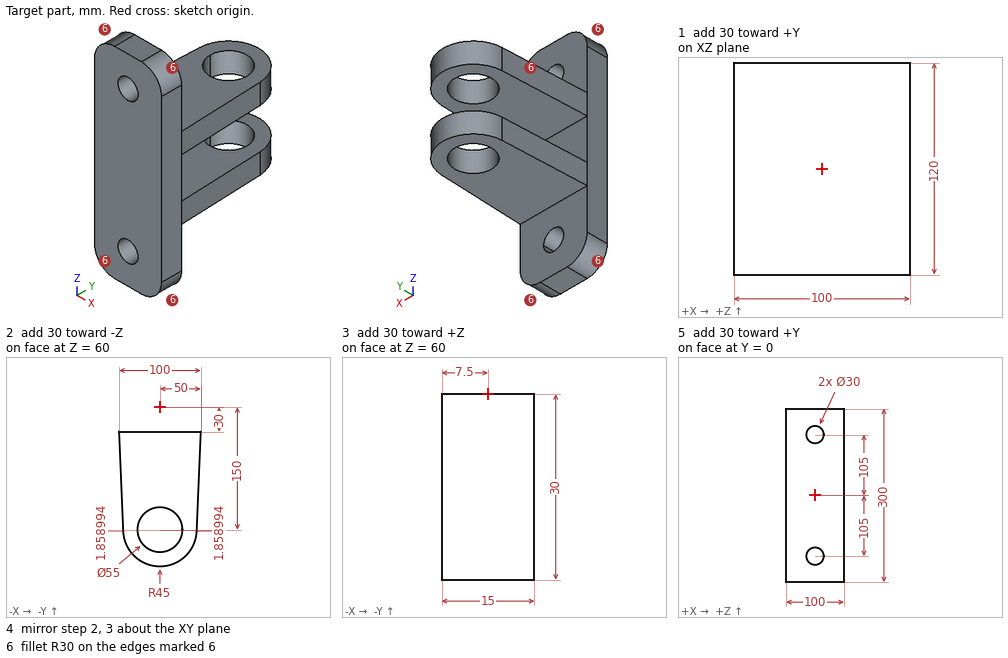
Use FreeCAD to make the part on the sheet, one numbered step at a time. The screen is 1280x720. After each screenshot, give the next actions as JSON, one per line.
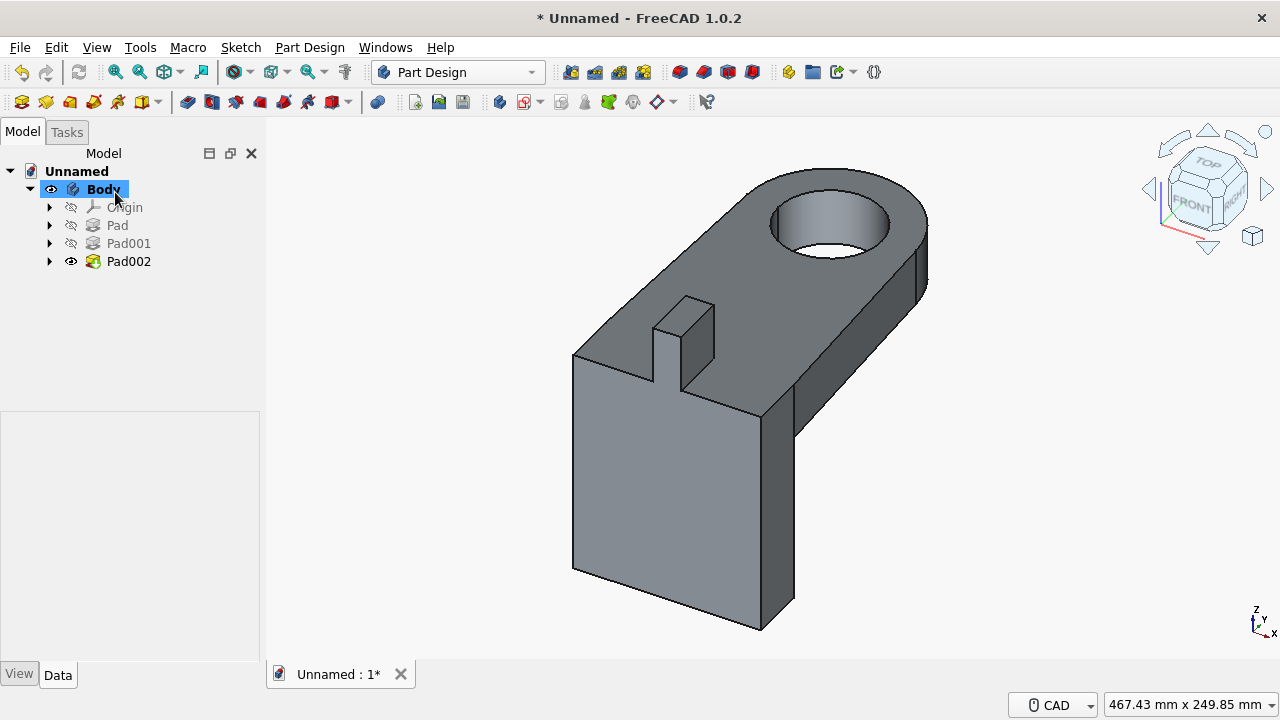
{"action": "key", "text": "v f"}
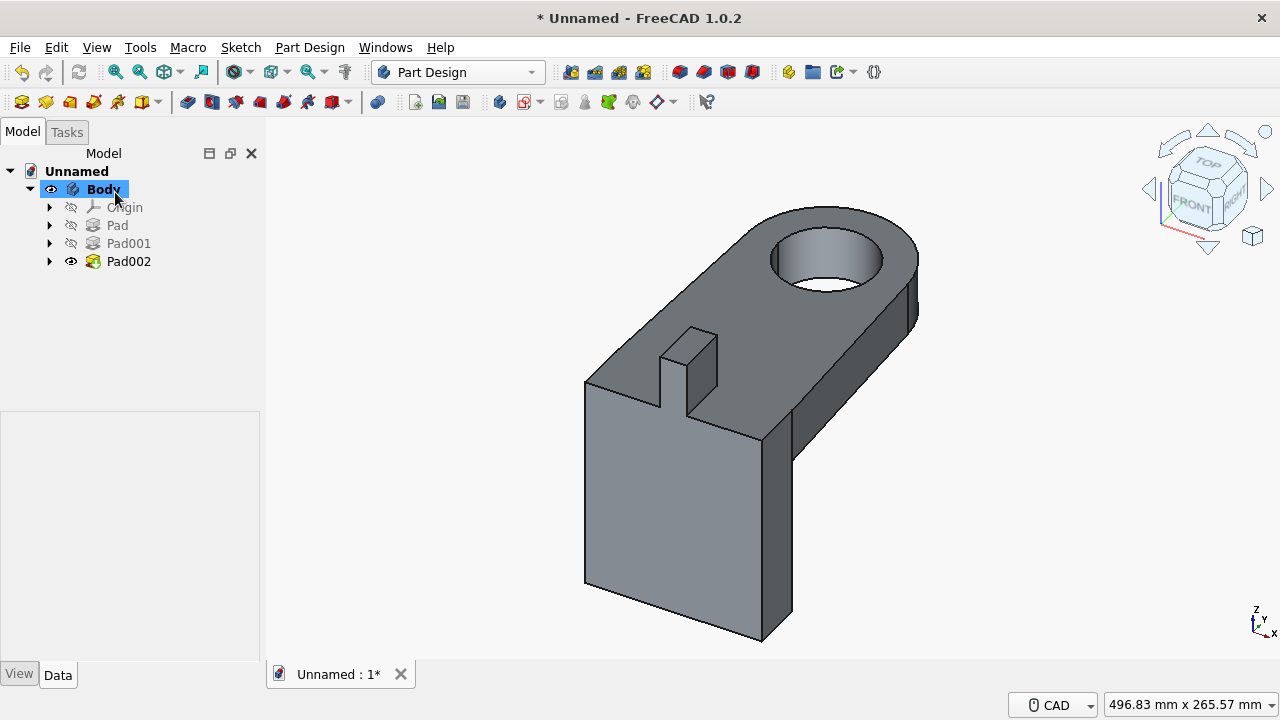
{"action": "left_click", "coordinate": [116, 243]}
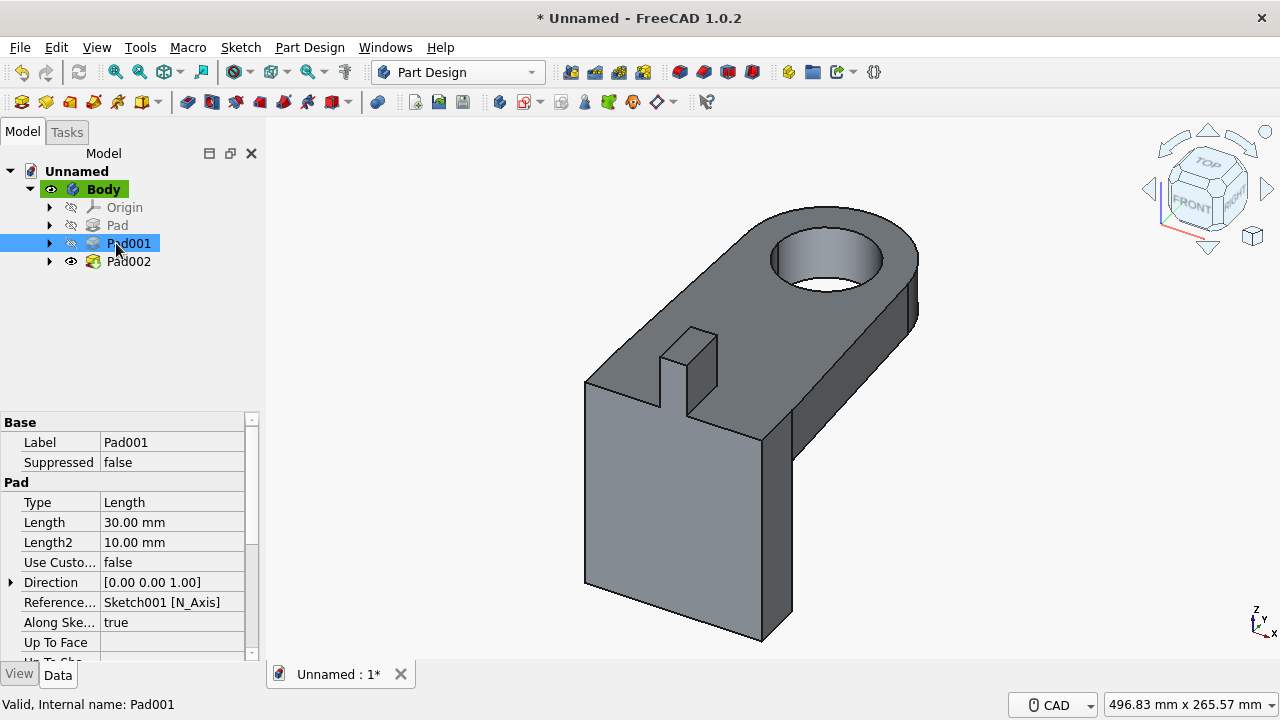
{"action": "left_click", "coordinate": [116, 261], "text": "ctrl"}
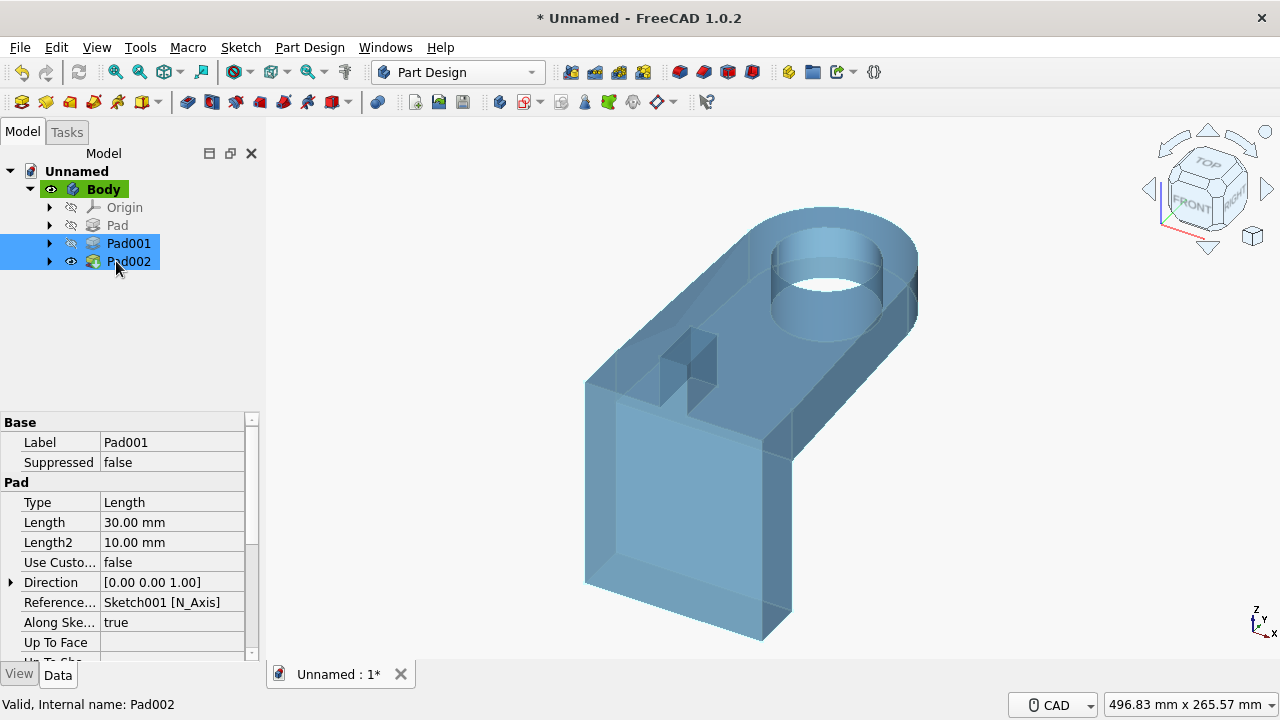
{"action": "left_click", "coordinate": [572, 72]}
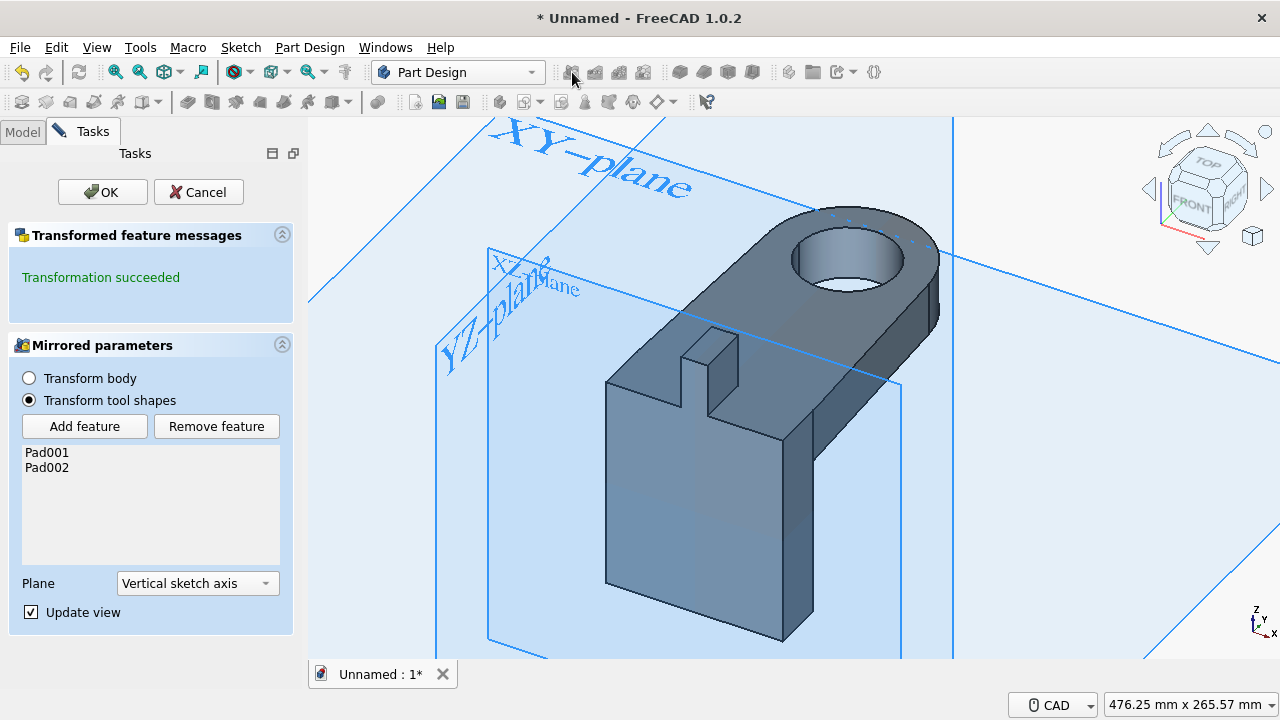
{"action": "left_click", "coordinate": [198, 584]}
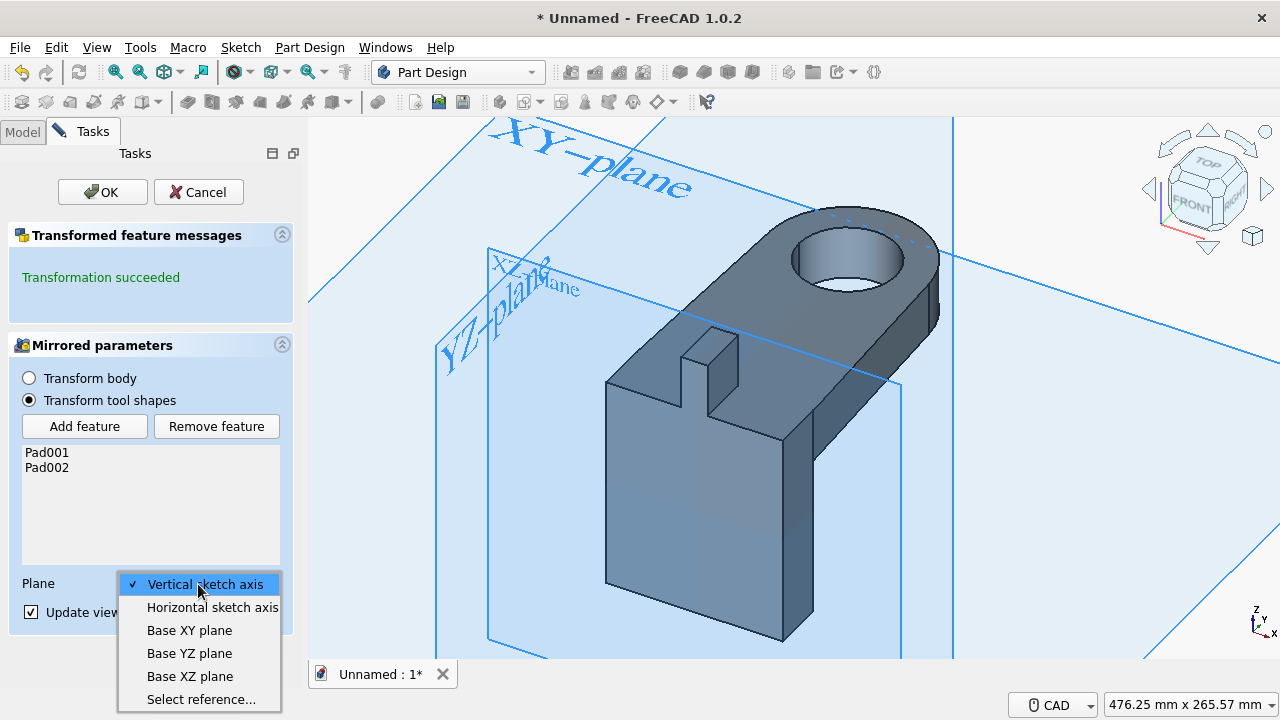
{"action": "left_click", "coordinate": [198, 630]}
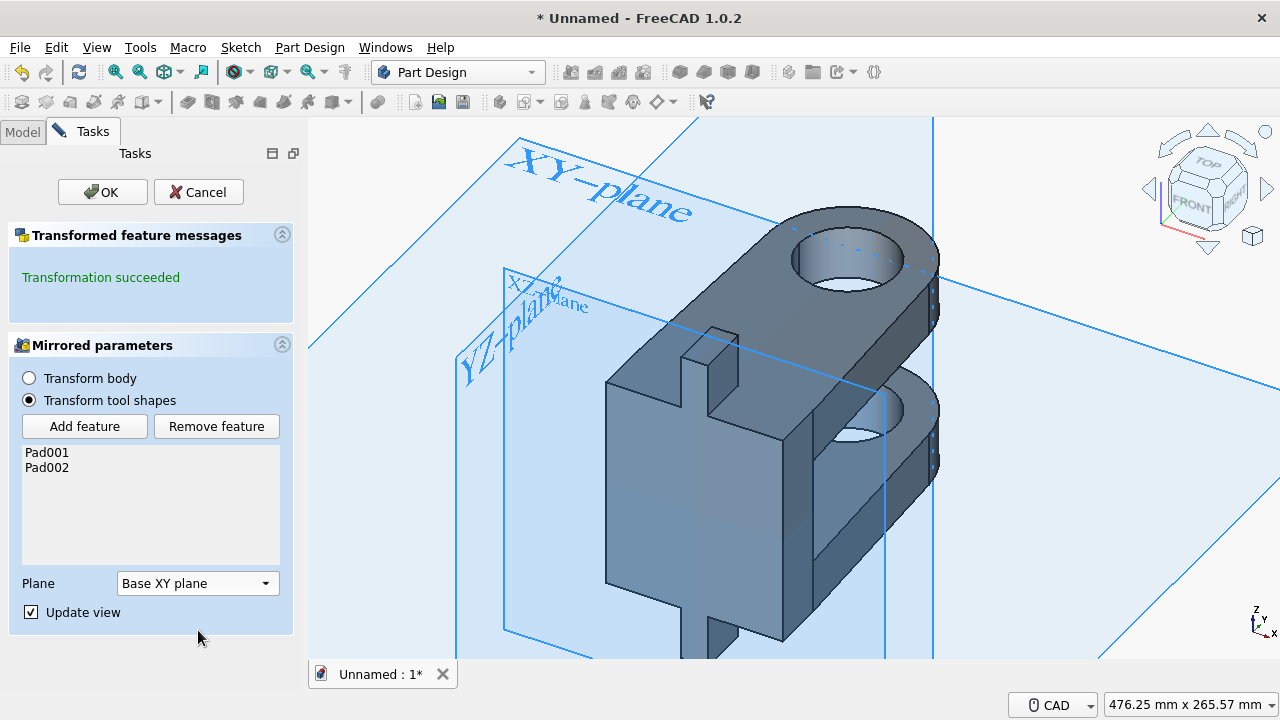
{"action": "left_click", "coordinate": [103, 192]}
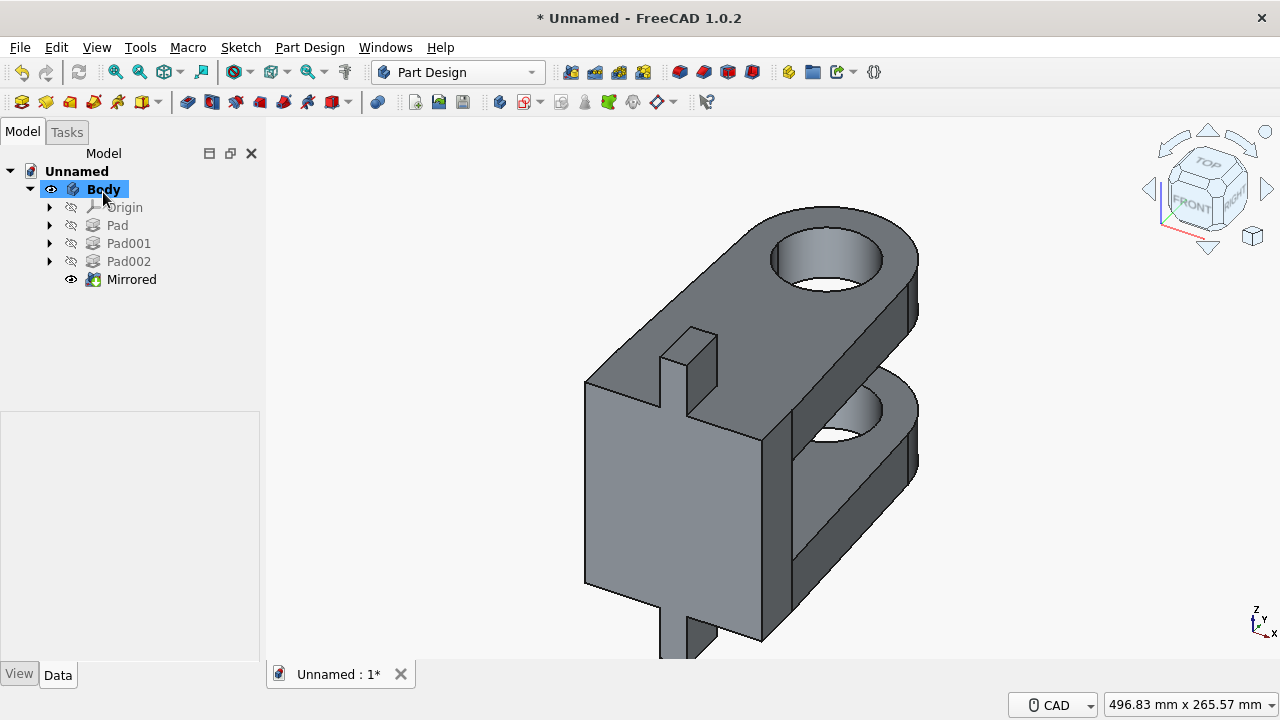
{"action": "key", "text": "v f"}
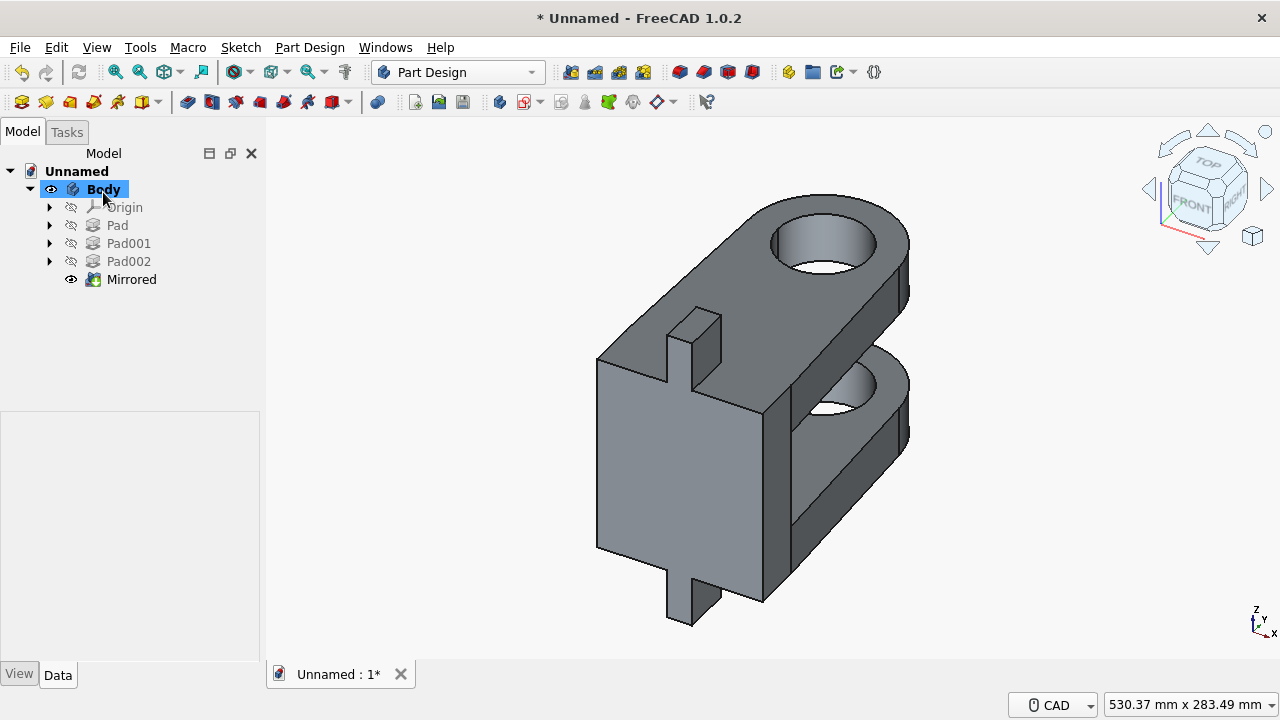
{"action": "left_click", "coordinate": [680, 480]}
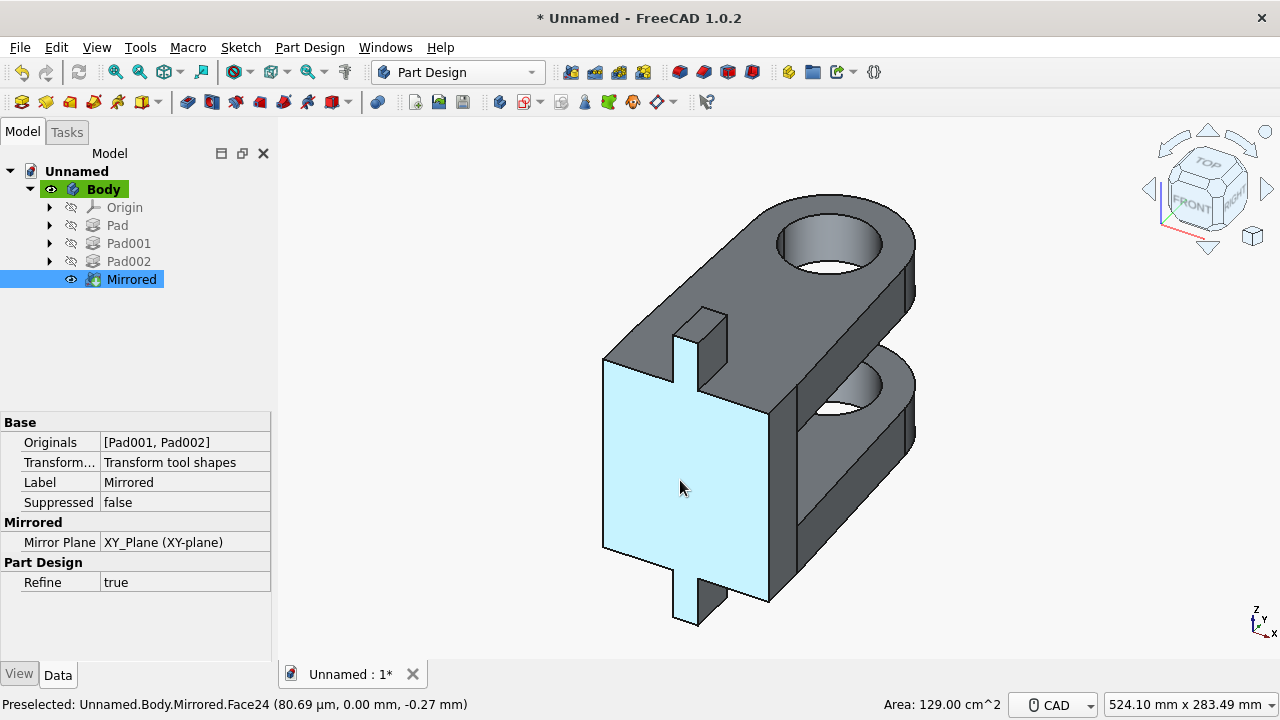
{"action": "left_click", "coordinate": [524, 102]}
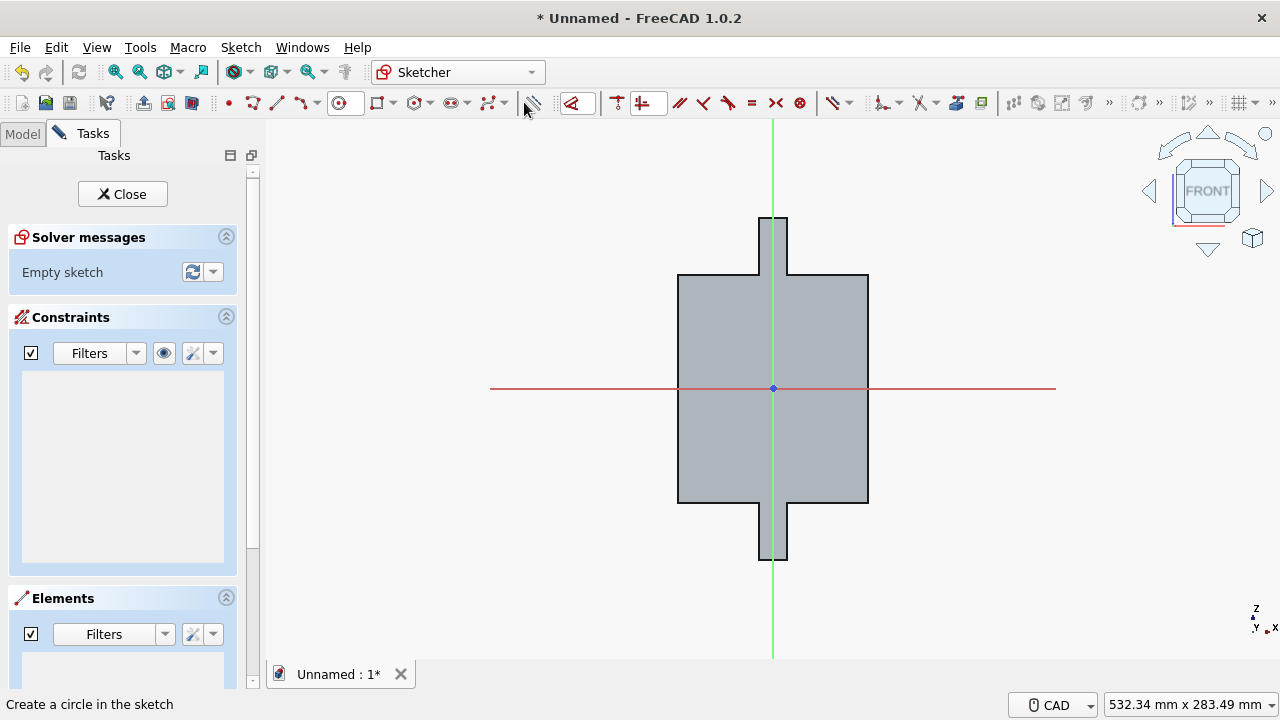
{"action": "scroll", "coordinate": [621, 389], "scroll_direction": "down", "scroll_amount": 3}